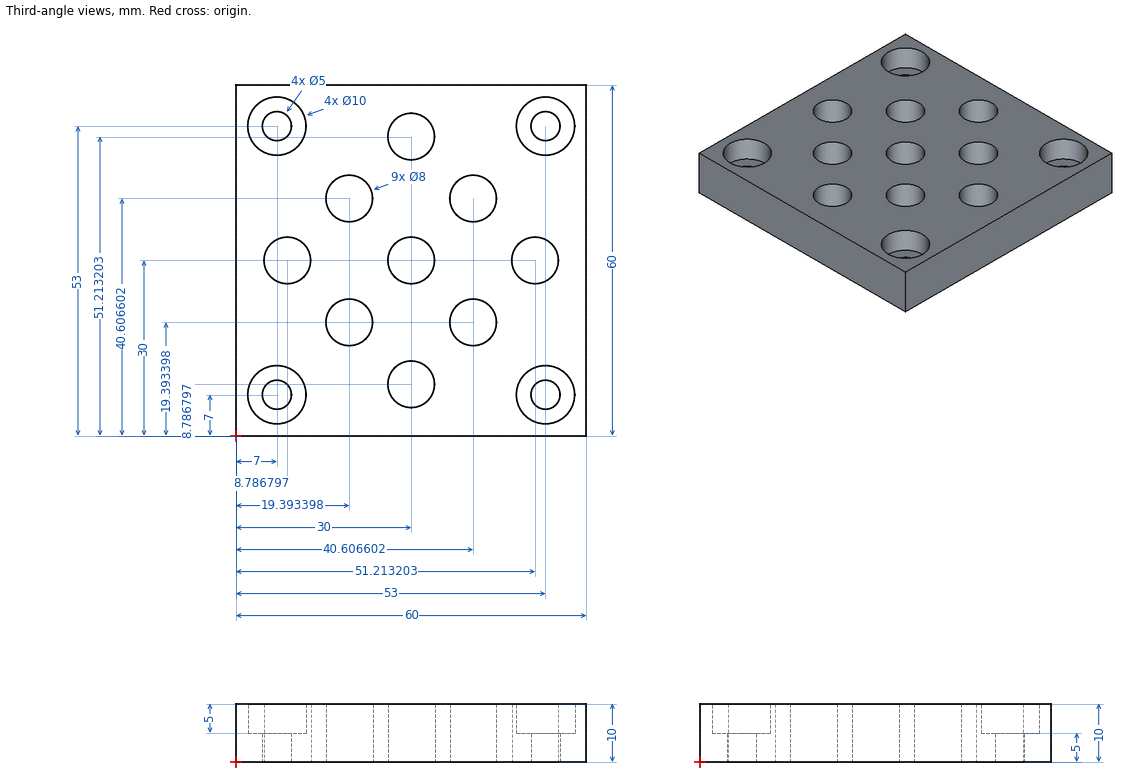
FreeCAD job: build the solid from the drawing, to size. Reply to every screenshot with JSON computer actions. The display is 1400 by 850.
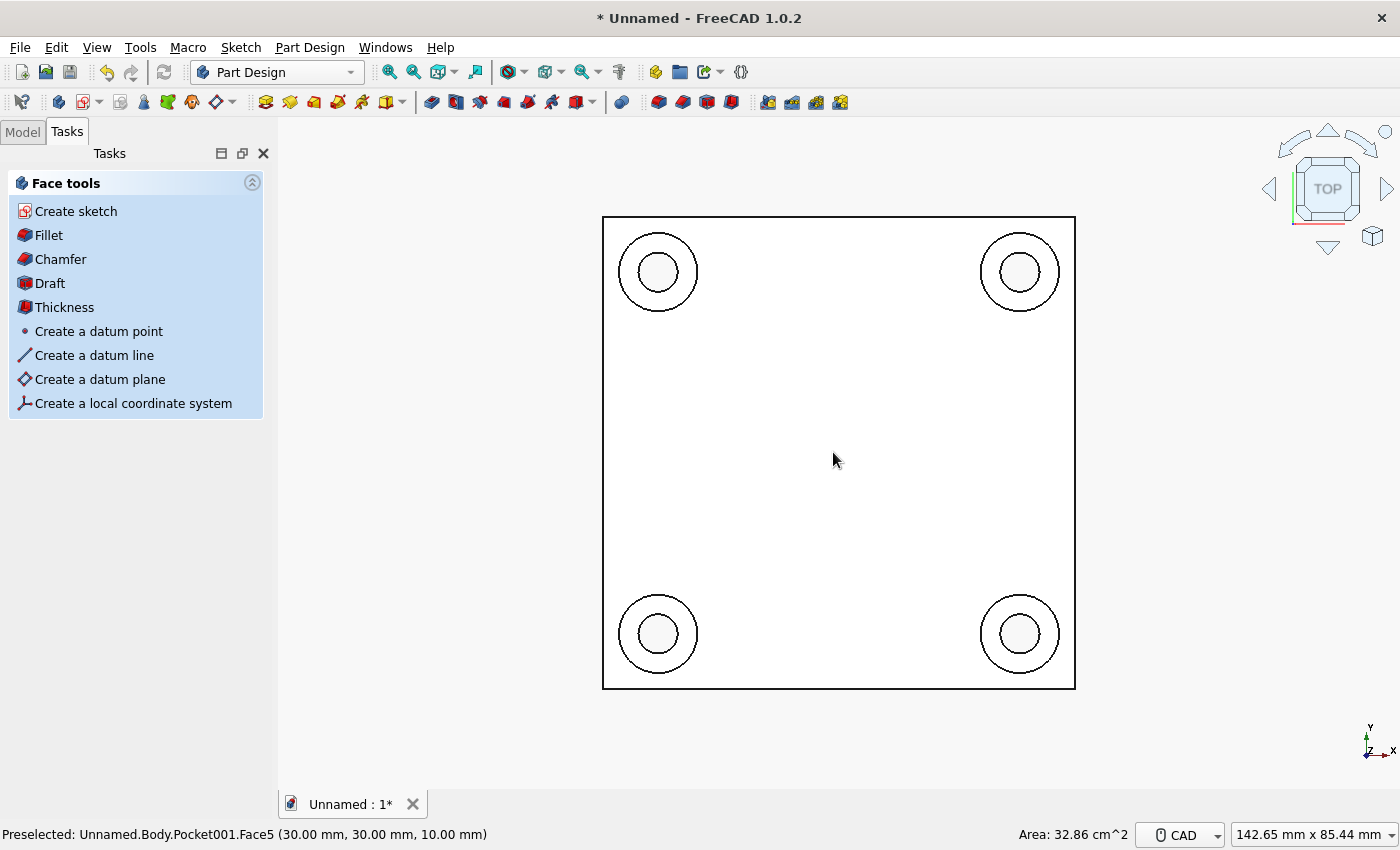
{"action": "left_click", "coordinate": [84, 102]}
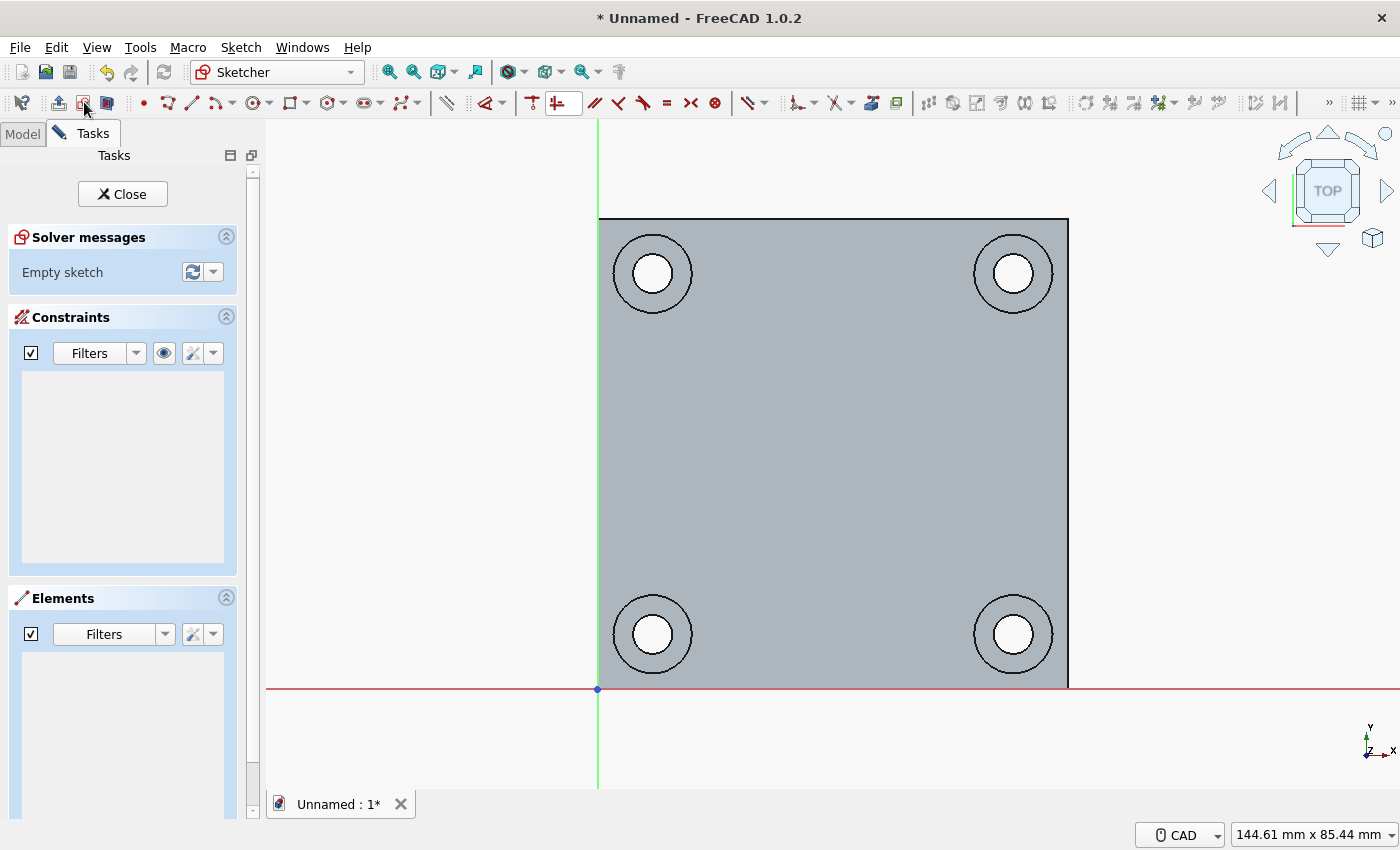
{"action": "left_click", "coordinate": [254, 104]}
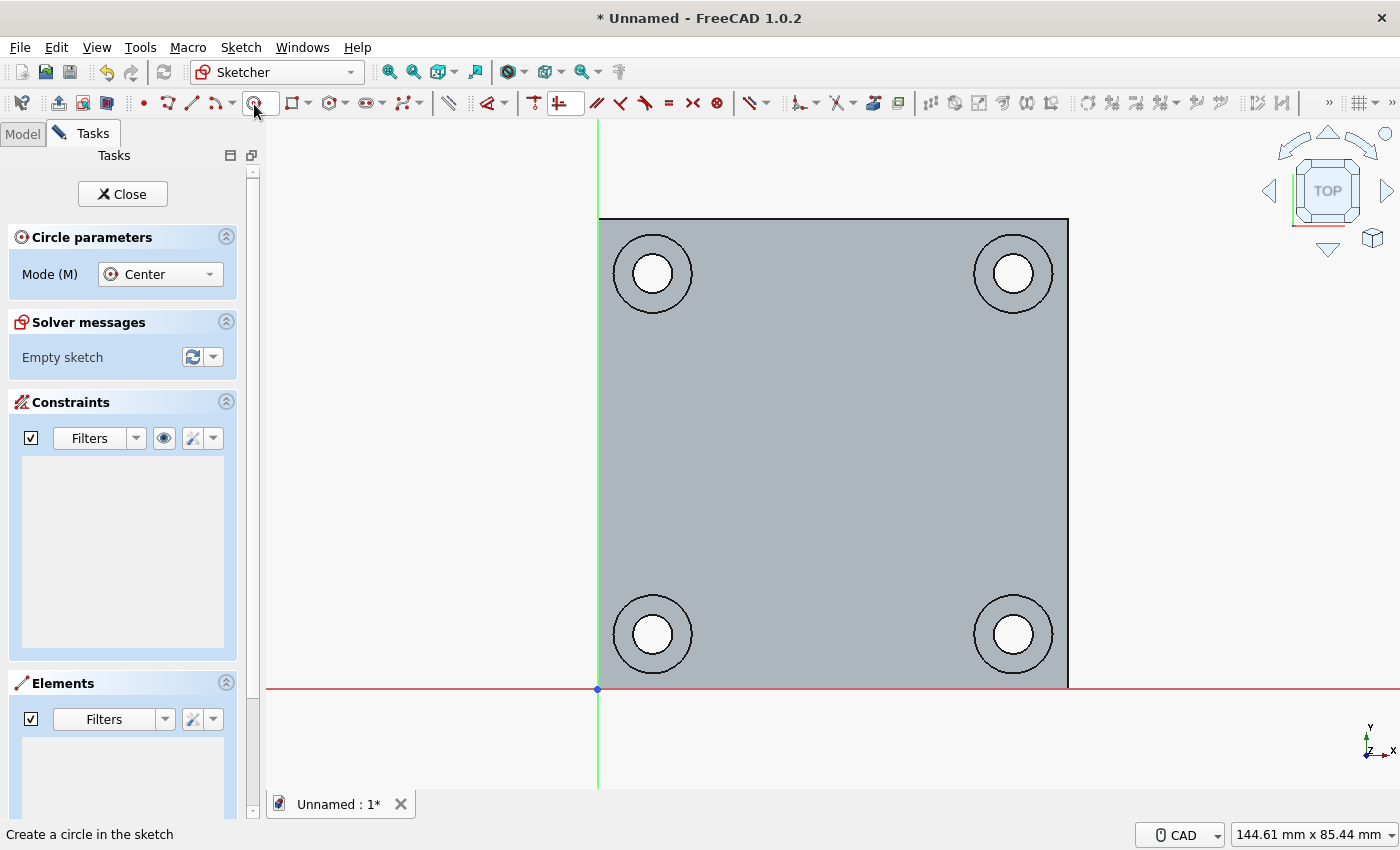
{"action": "left_click", "coordinate": [750, 371]}
{"action": "left_click", "coordinate": [772, 349]}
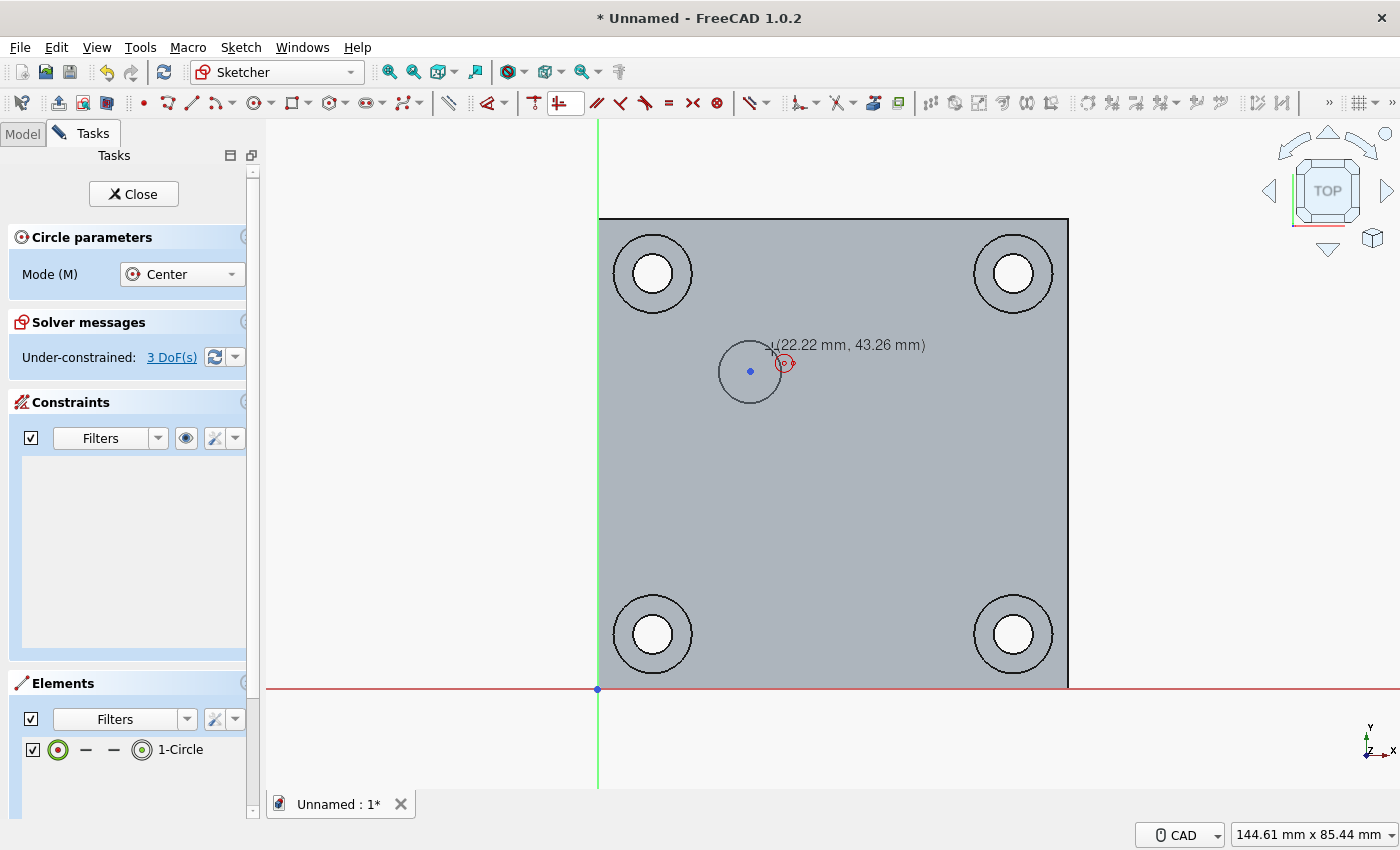
{"action": "left_click", "coordinate": [833, 288]}
{"action": "left_click", "coordinate": [855, 265]}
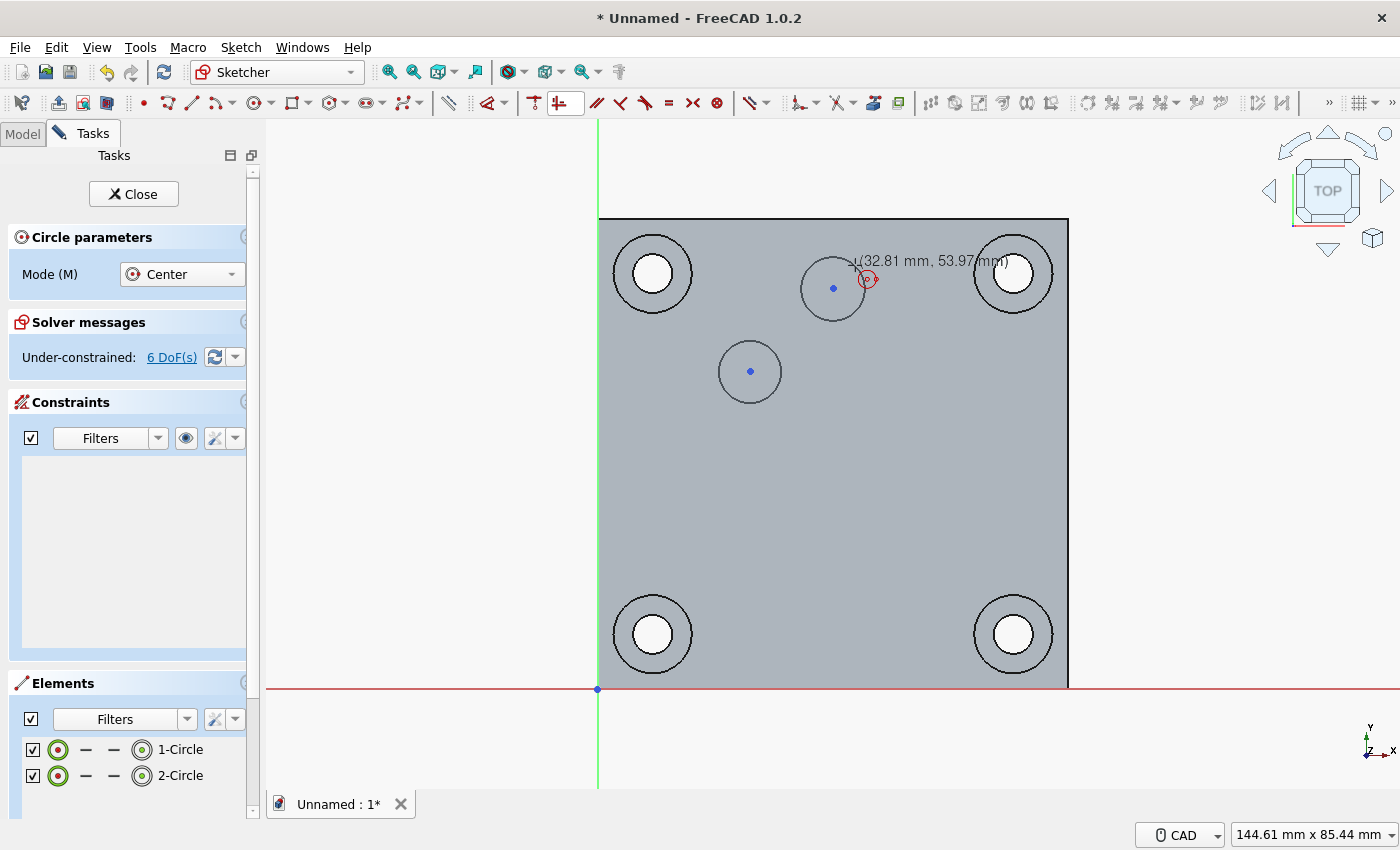
{"action": "left_click", "coordinate": [916, 371]}
{"action": "left_click", "coordinate": [938, 349]}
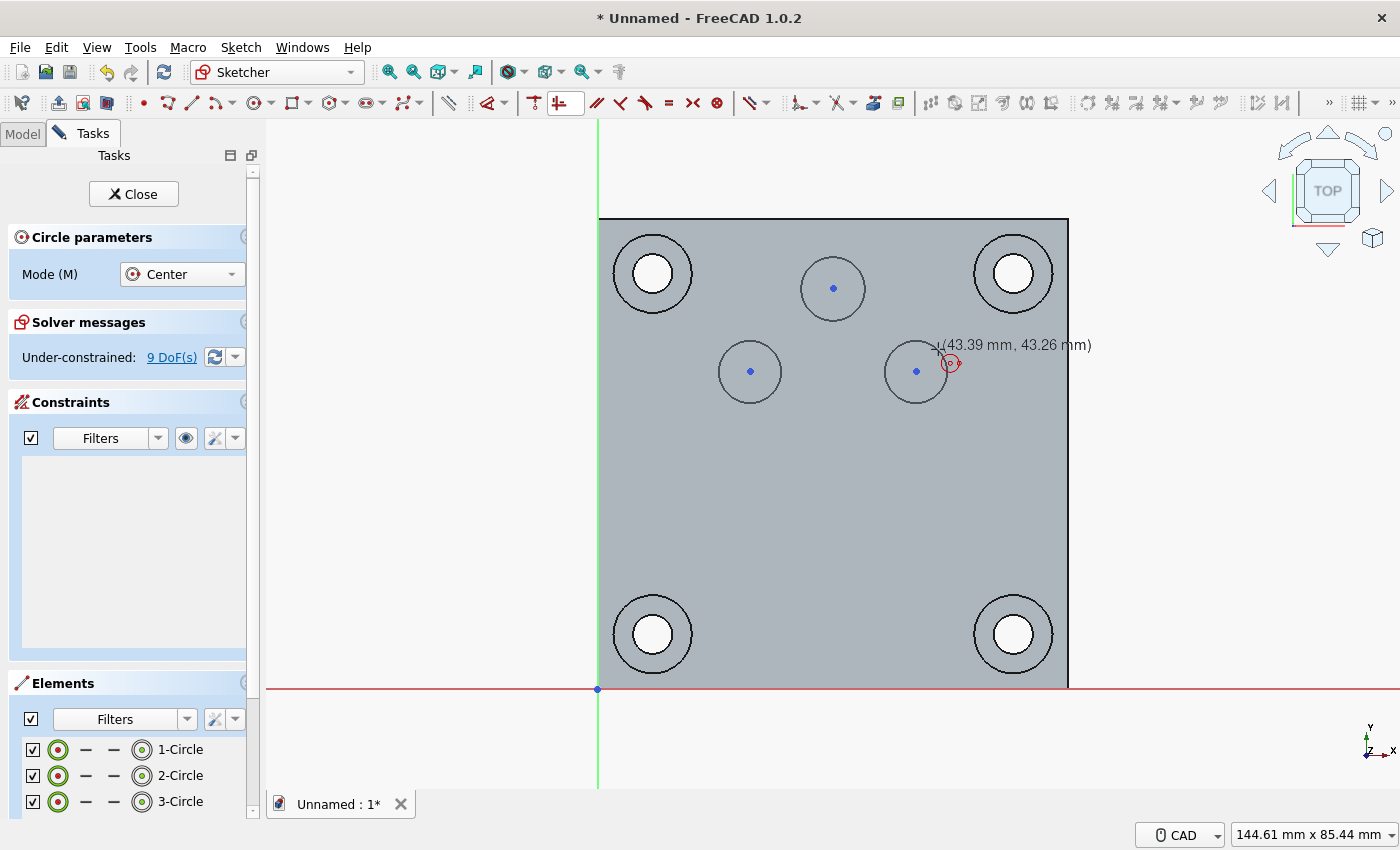
{"action": "left_click", "coordinate": [999, 454]}
{"action": "left_click", "coordinate": [1022, 432]}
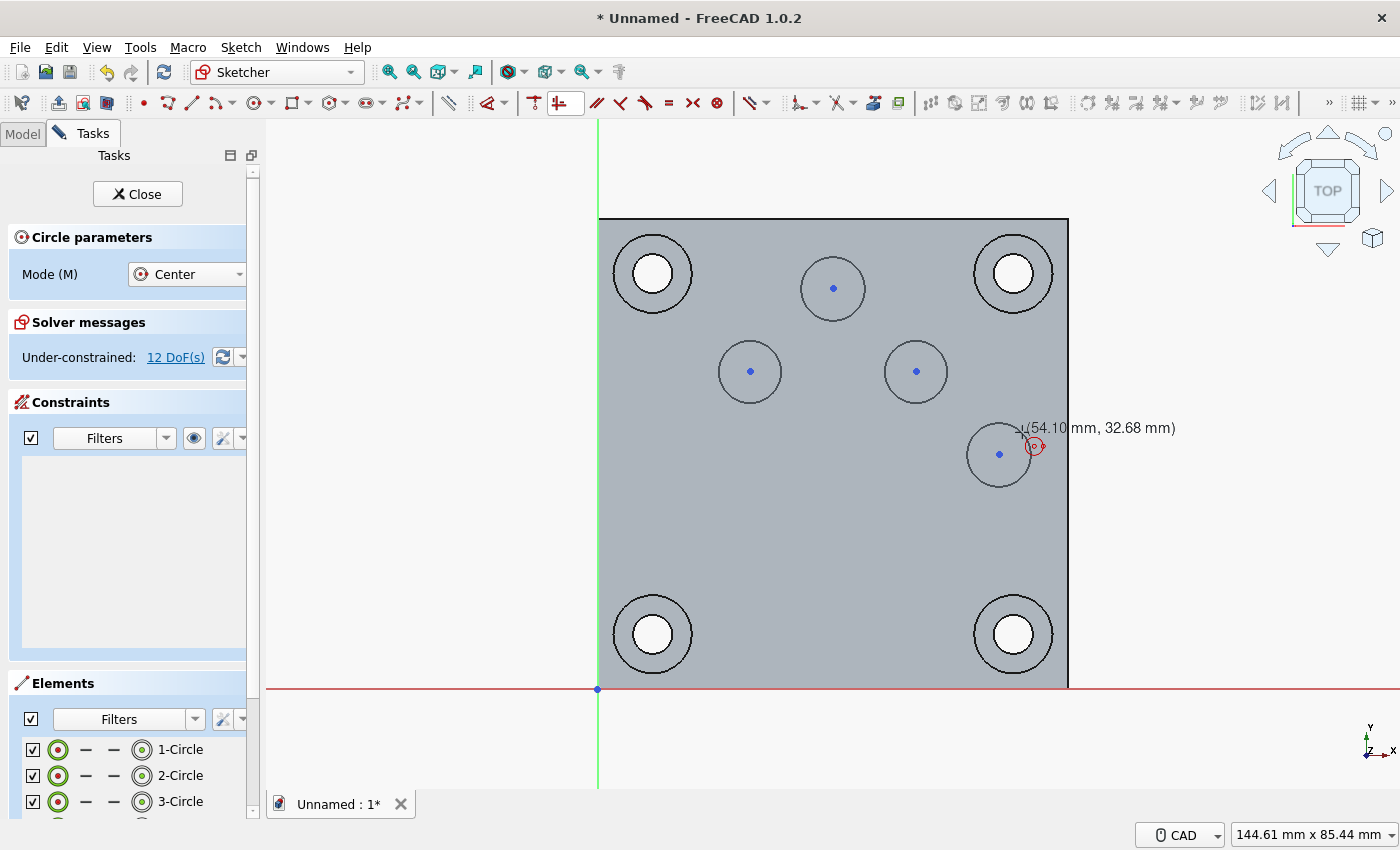
{"action": "left_click", "coordinate": [916, 537]}
{"action": "left_click", "coordinate": [938, 515]}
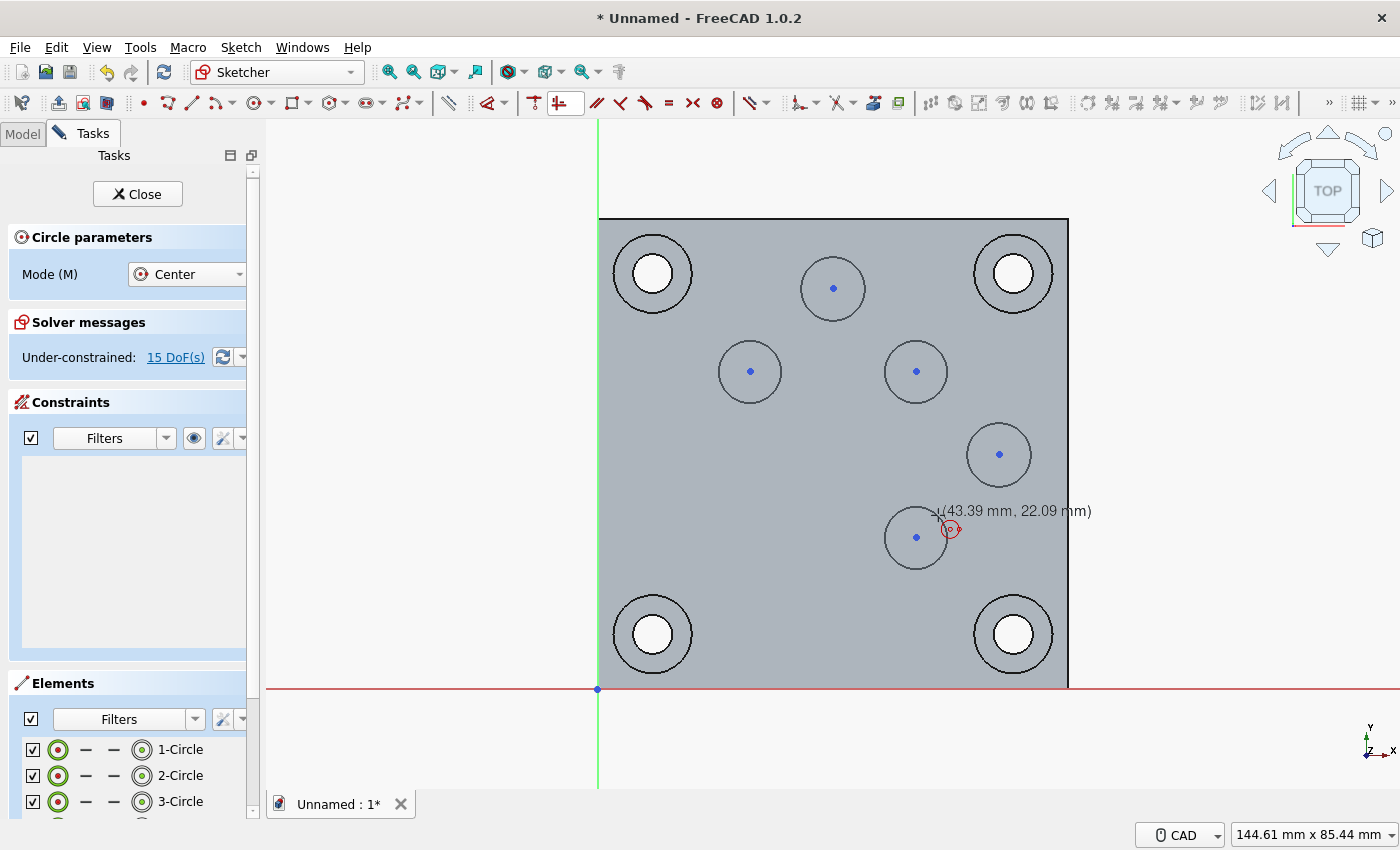
{"action": "left_click", "coordinate": [750, 537]}
{"action": "left_click", "coordinate": [772, 515]}